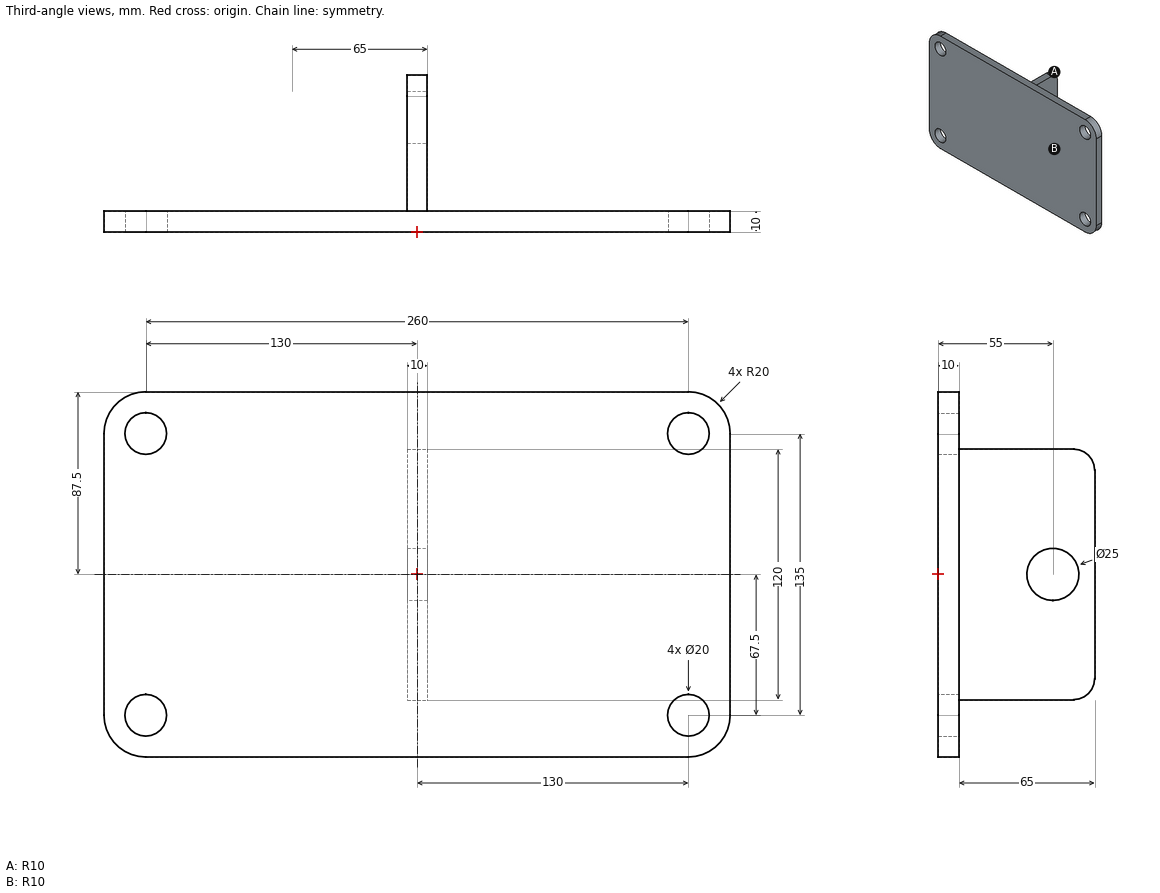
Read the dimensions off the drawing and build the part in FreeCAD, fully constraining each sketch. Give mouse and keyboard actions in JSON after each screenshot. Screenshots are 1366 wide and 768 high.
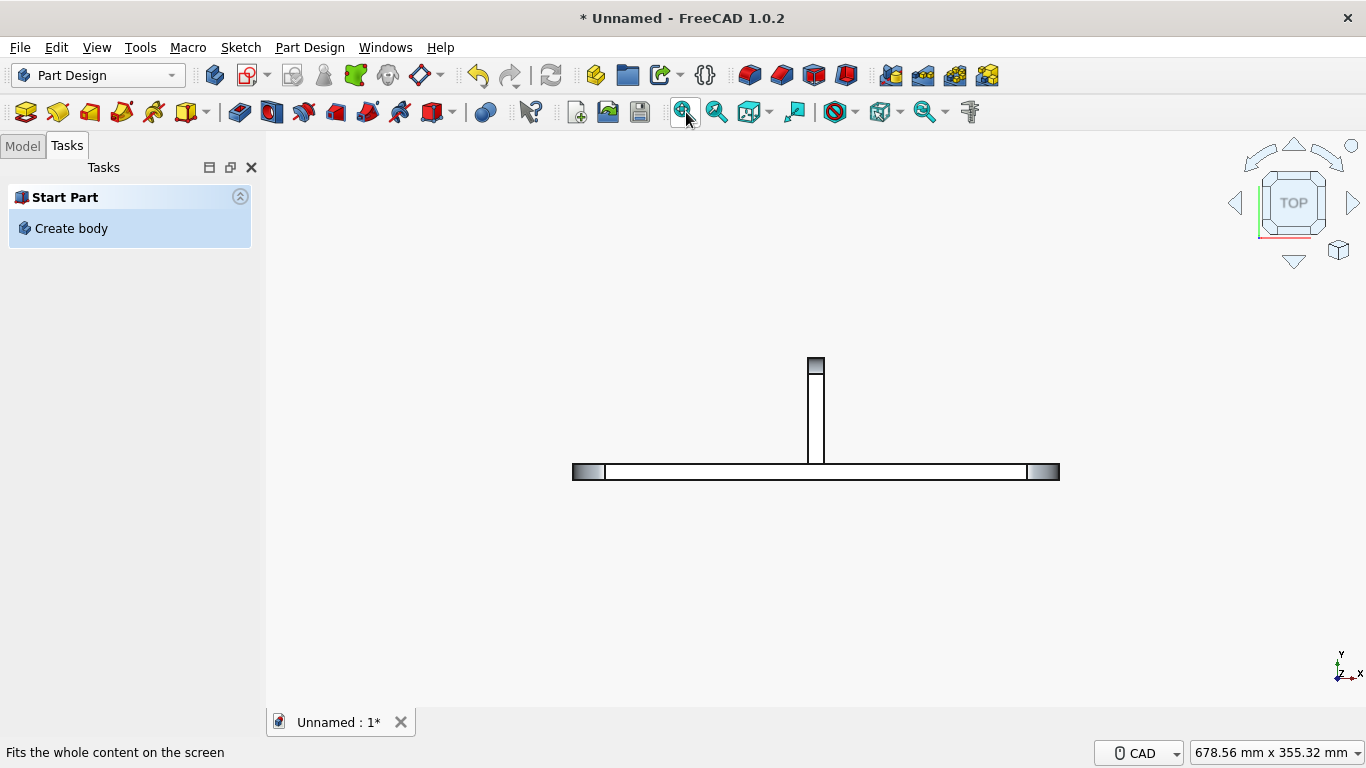
{"action": "scroll", "coordinate": [816, 357], "scroll_direction": "up", "scroll_amount": 5}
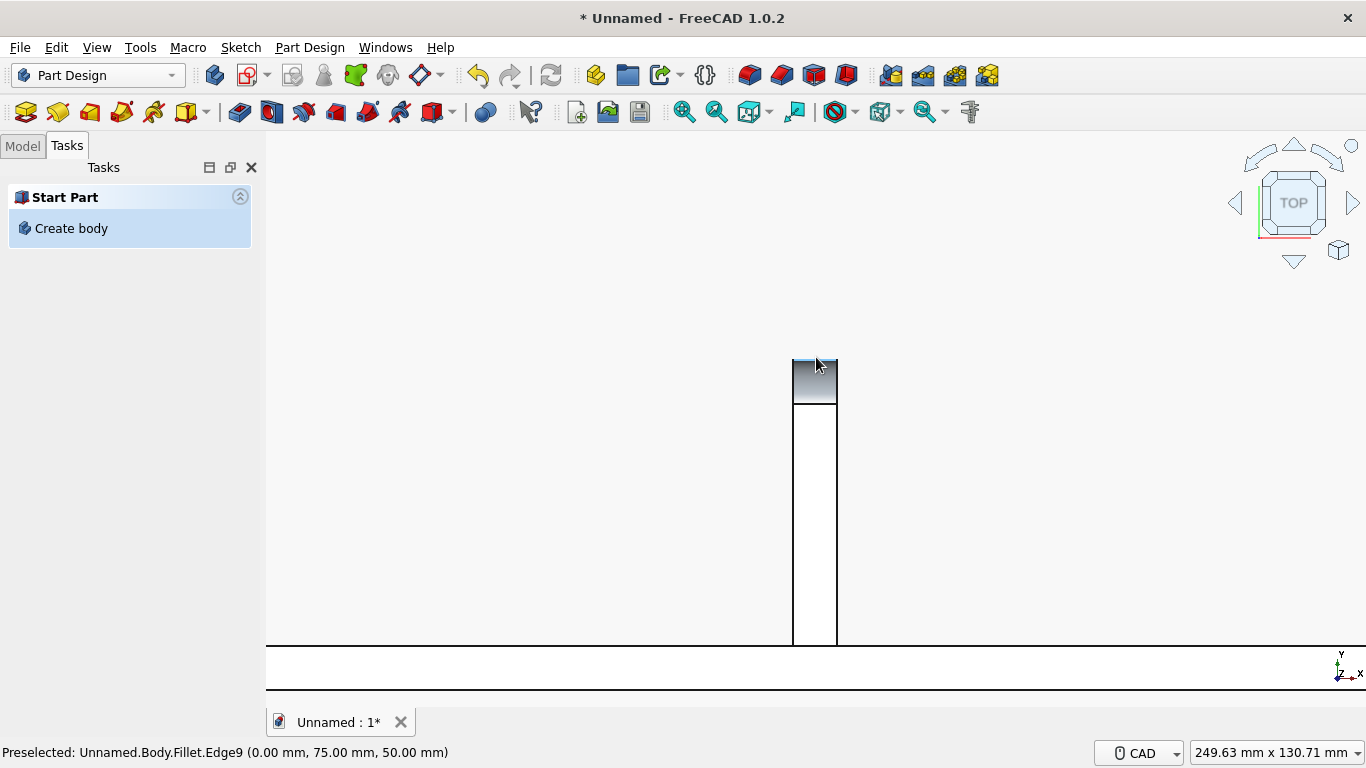
{"action": "left_click", "coordinate": [686, 112]}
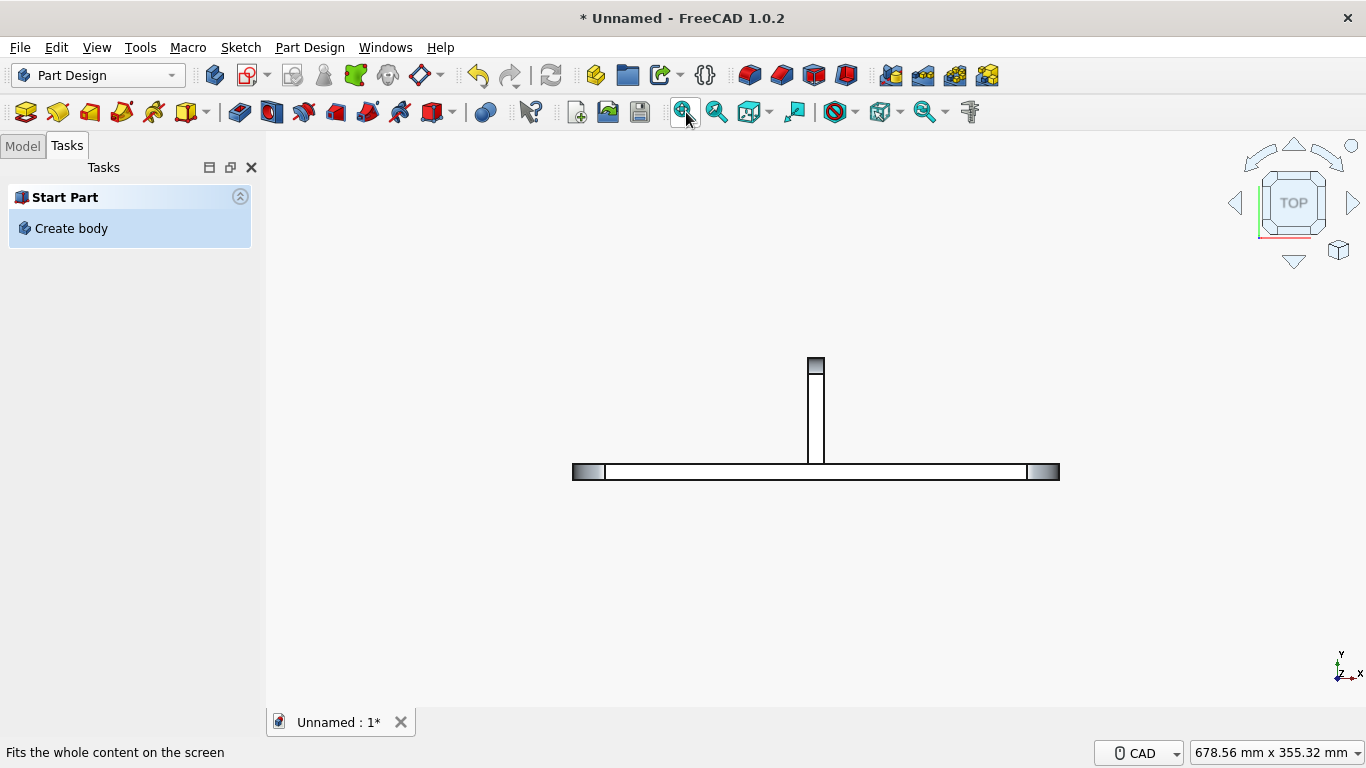
{"action": "key", "text": "1"}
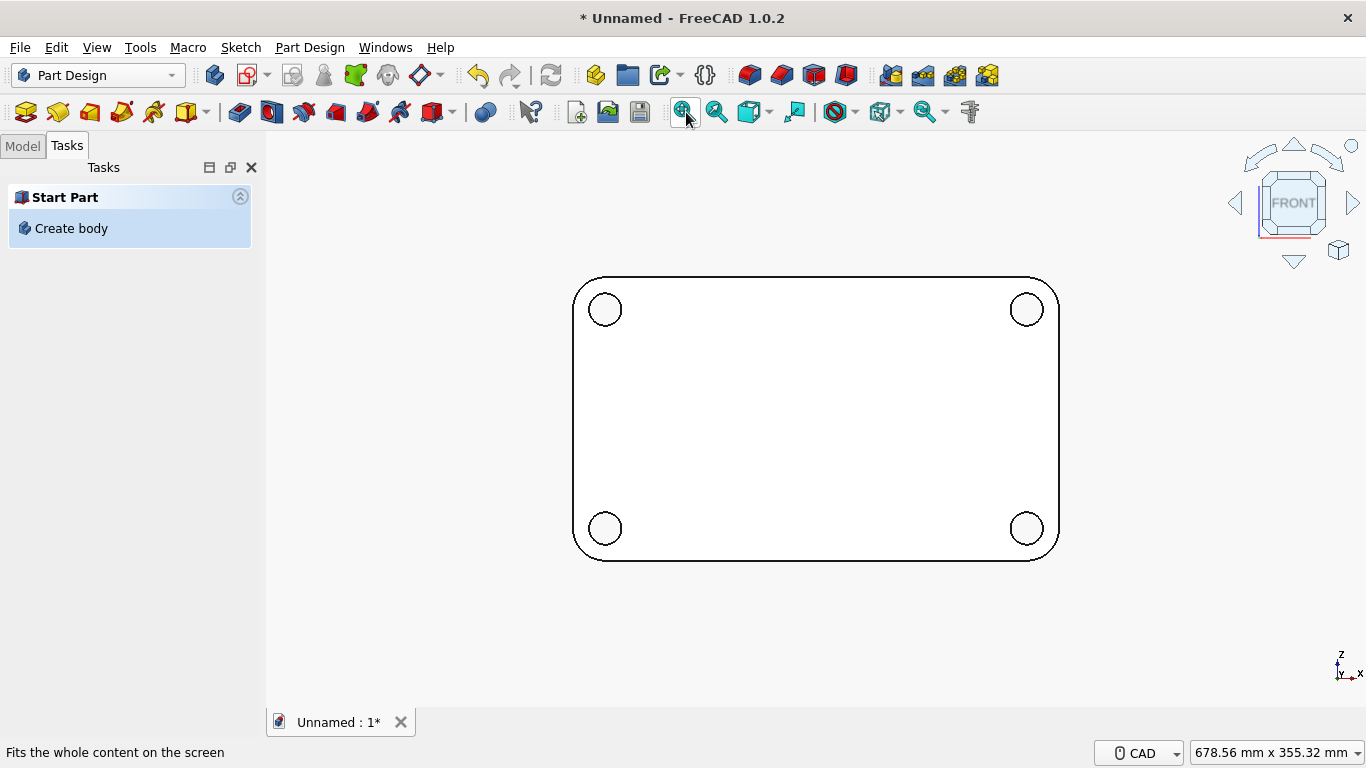
{"action": "scroll", "coordinate": [816, 515], "scroll_direction": "up", "scroll_amount": 5}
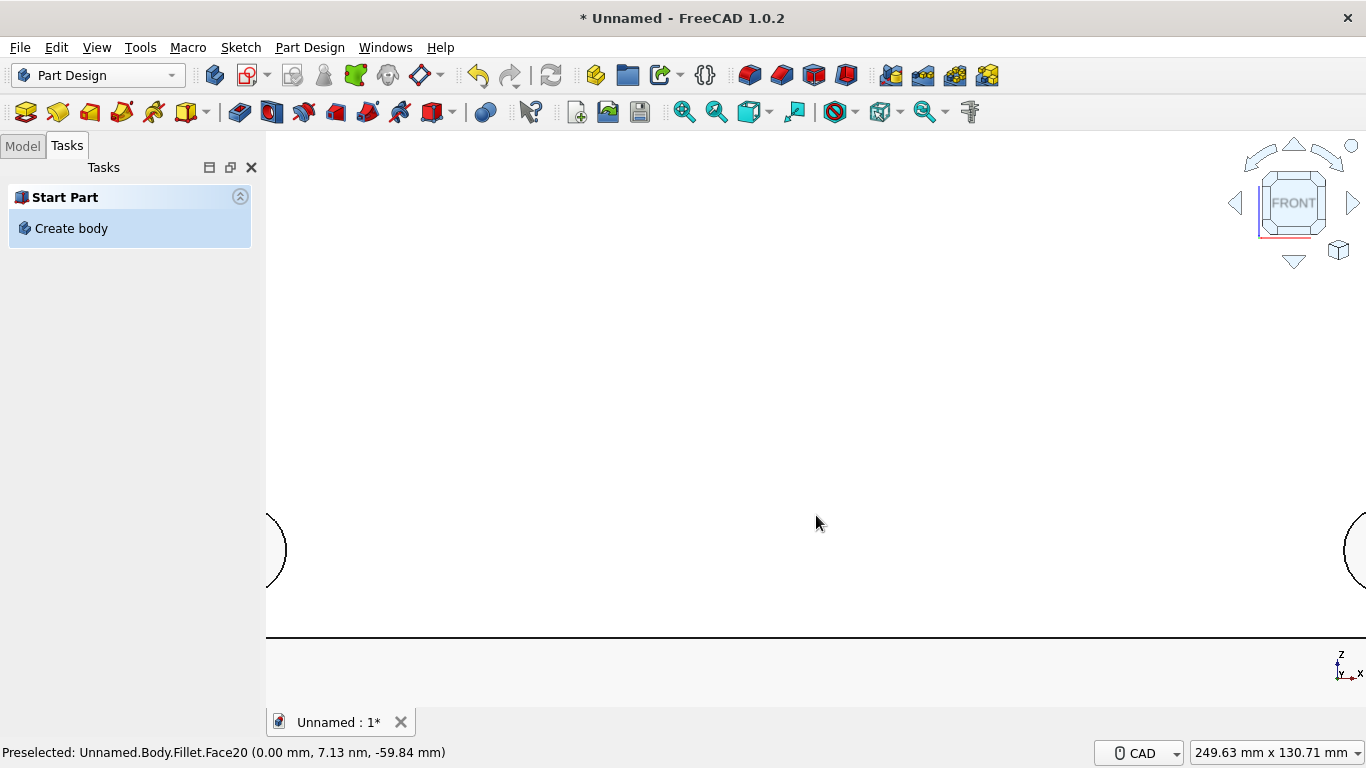
{"action": "left_click", "coordinate": [686, 112]}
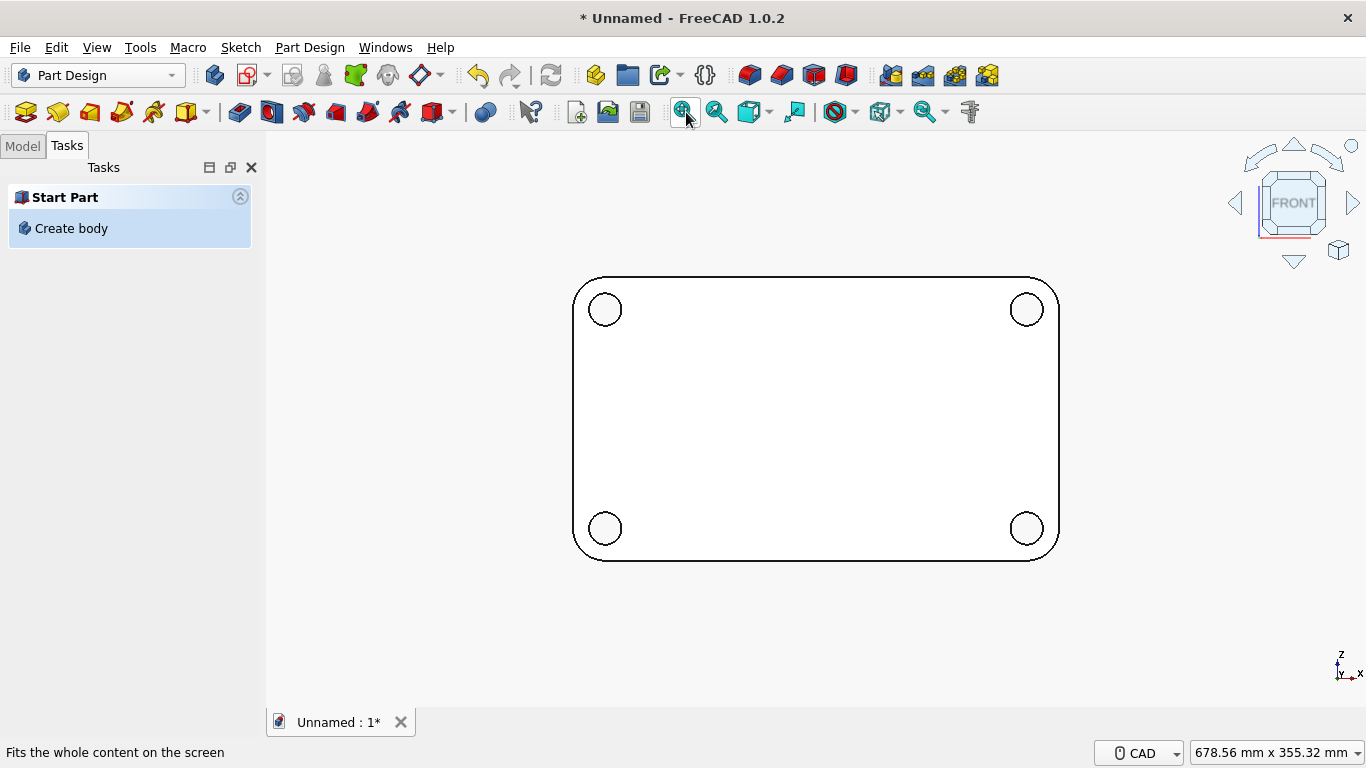
{"action": "key", "text": "3"}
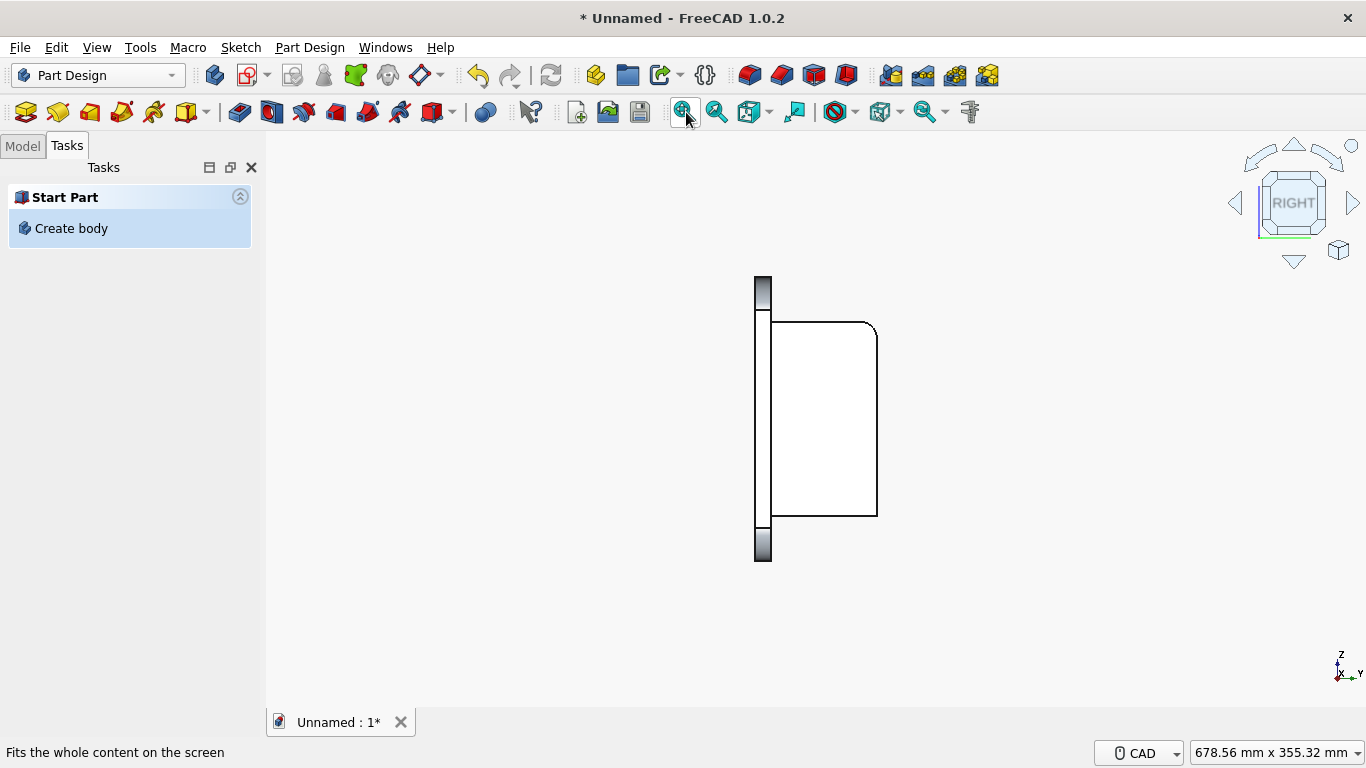
{"action": "scroll", "coordinate": [877, 515], "scroll_direction": "up", "scroll_amount": 5}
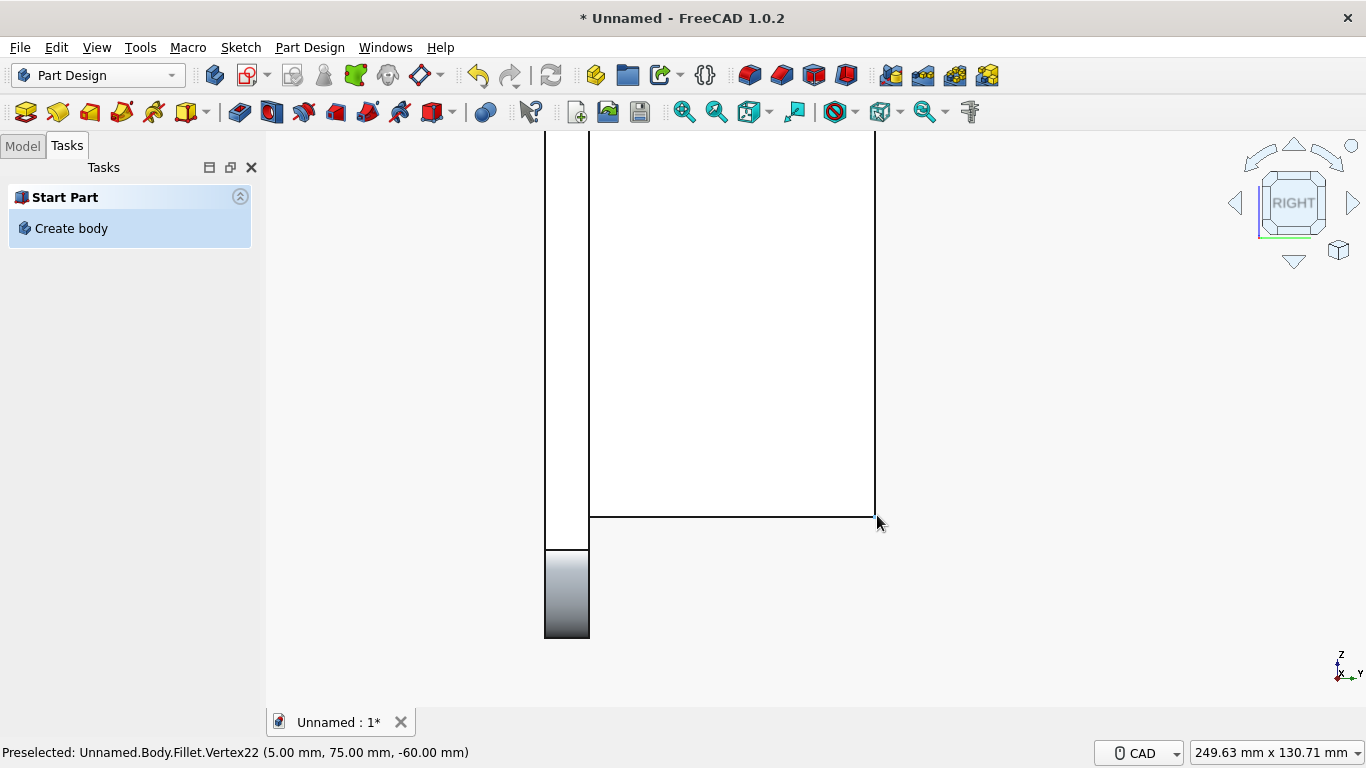
{"action": "left_click", "coordinate": [686, 112]}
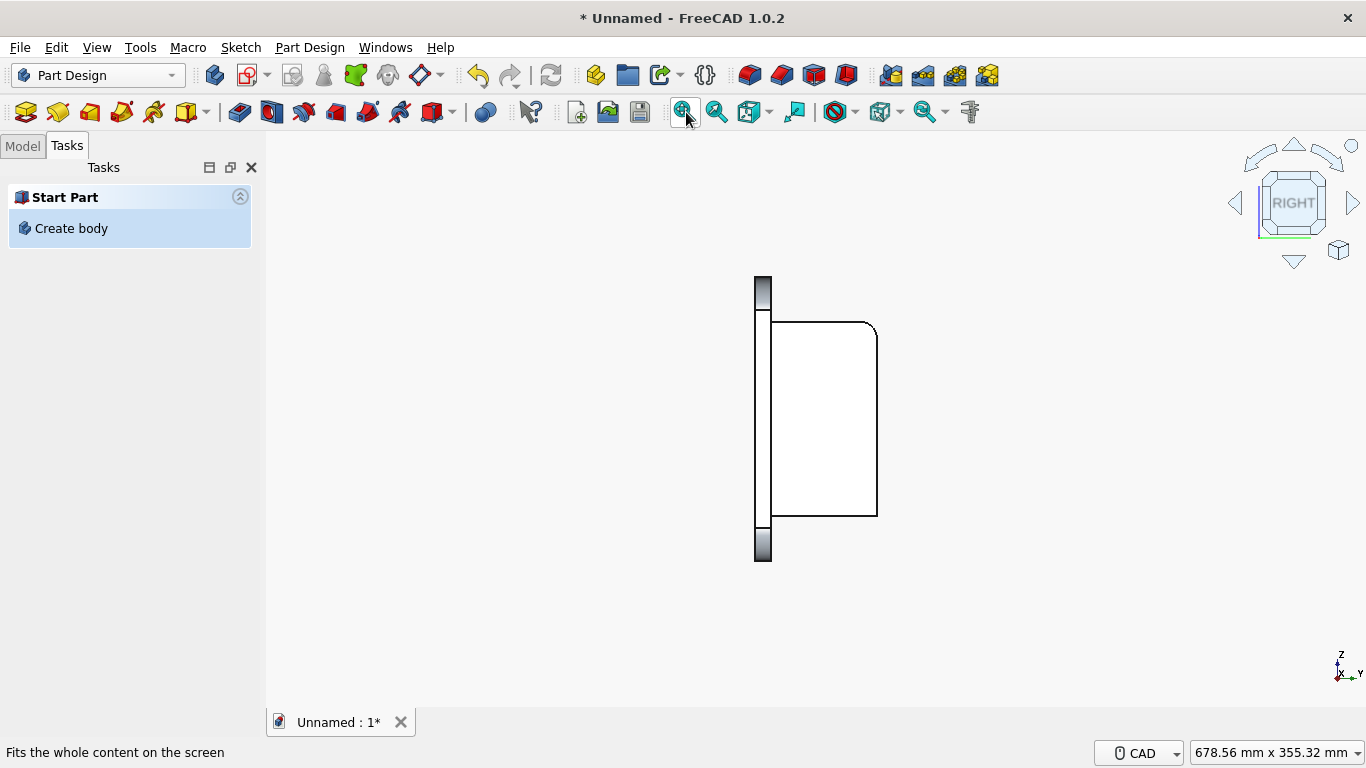
{"action": "key", "text": "5"}